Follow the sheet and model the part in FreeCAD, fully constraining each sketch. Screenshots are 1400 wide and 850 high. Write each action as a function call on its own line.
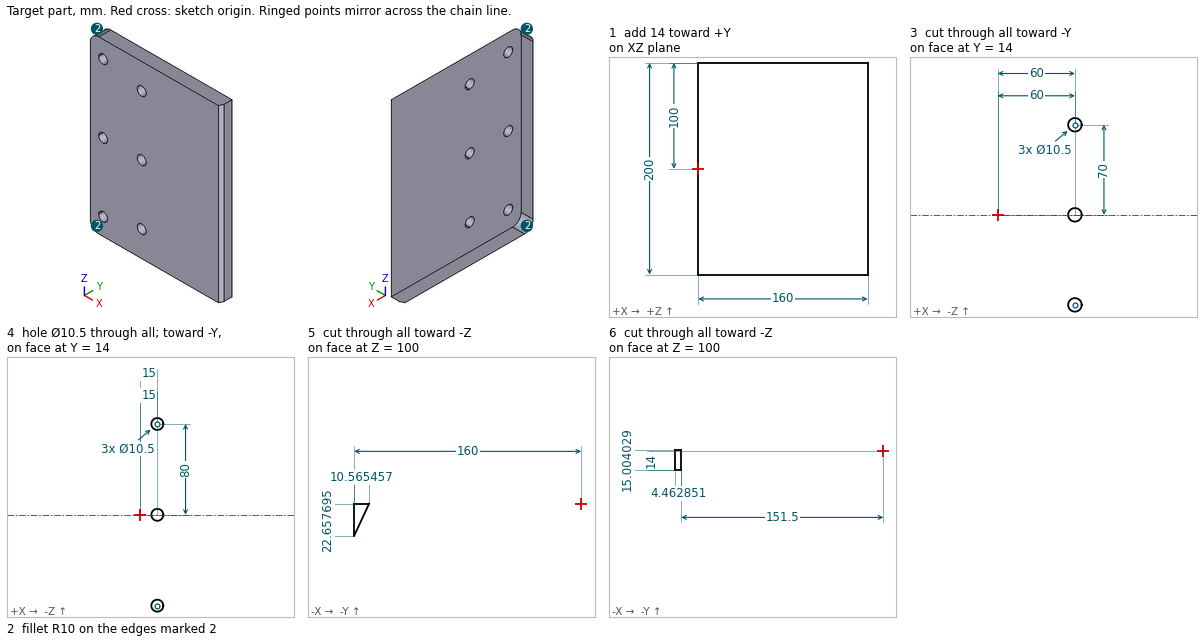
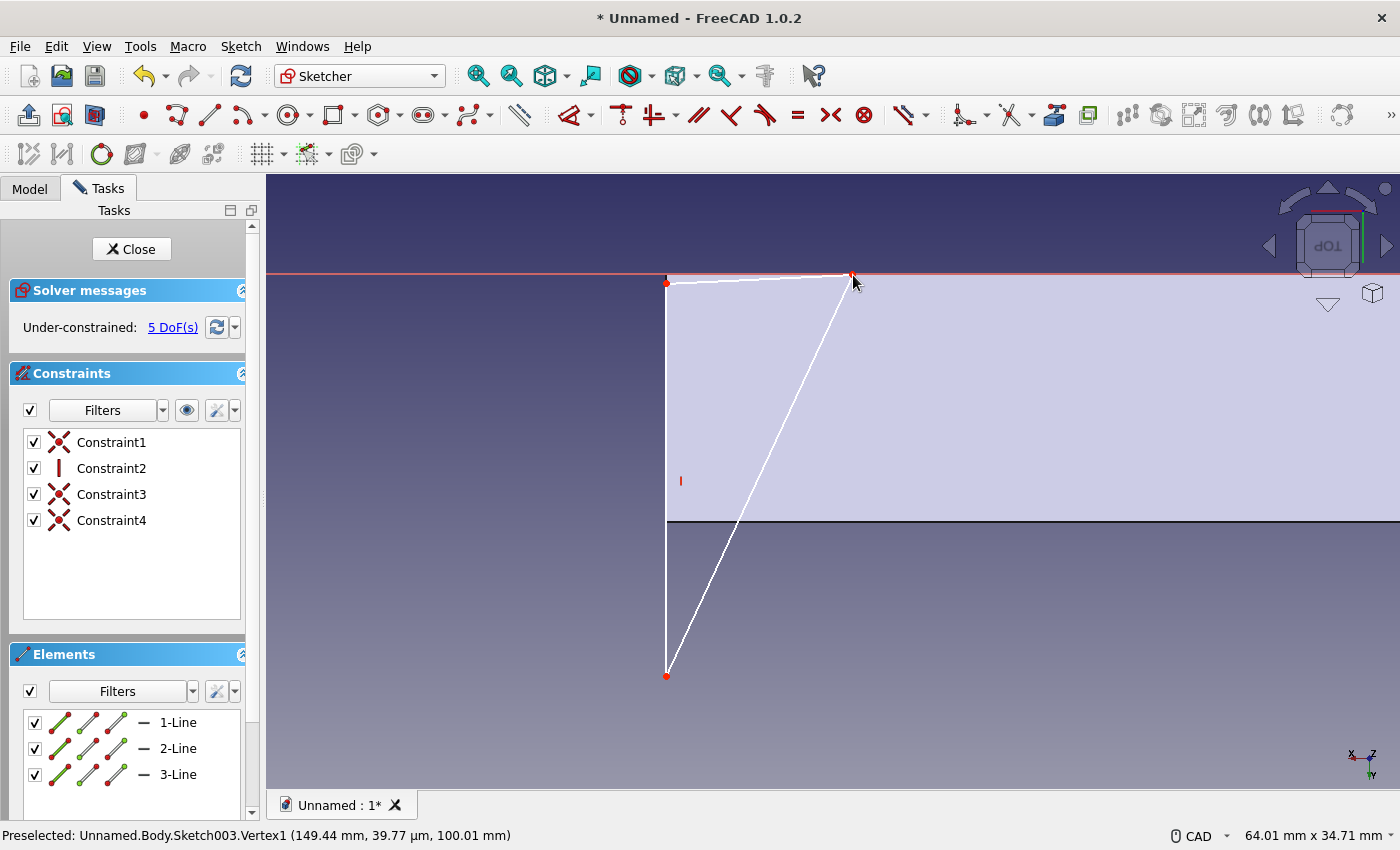
click(797, 278)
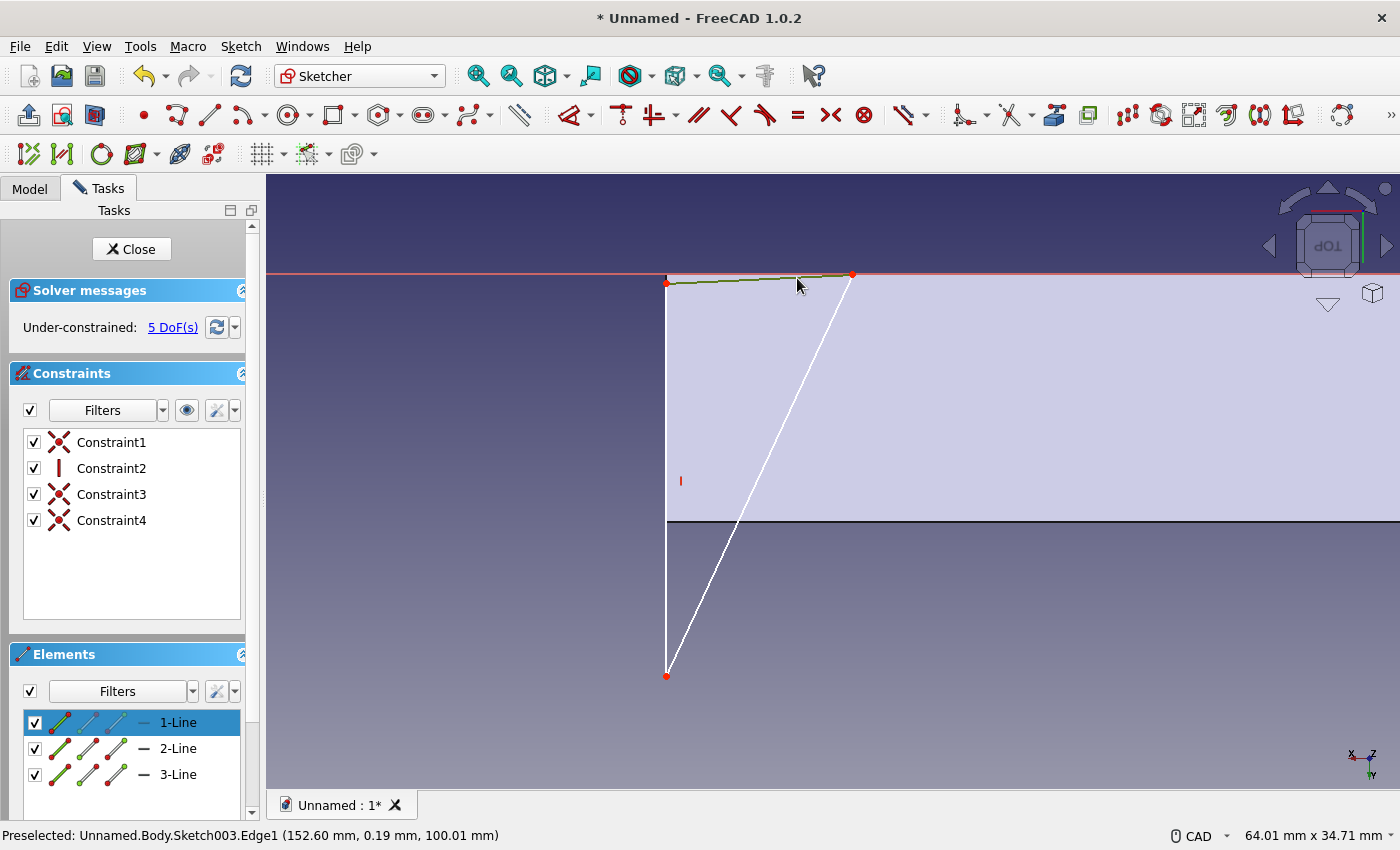
key(h)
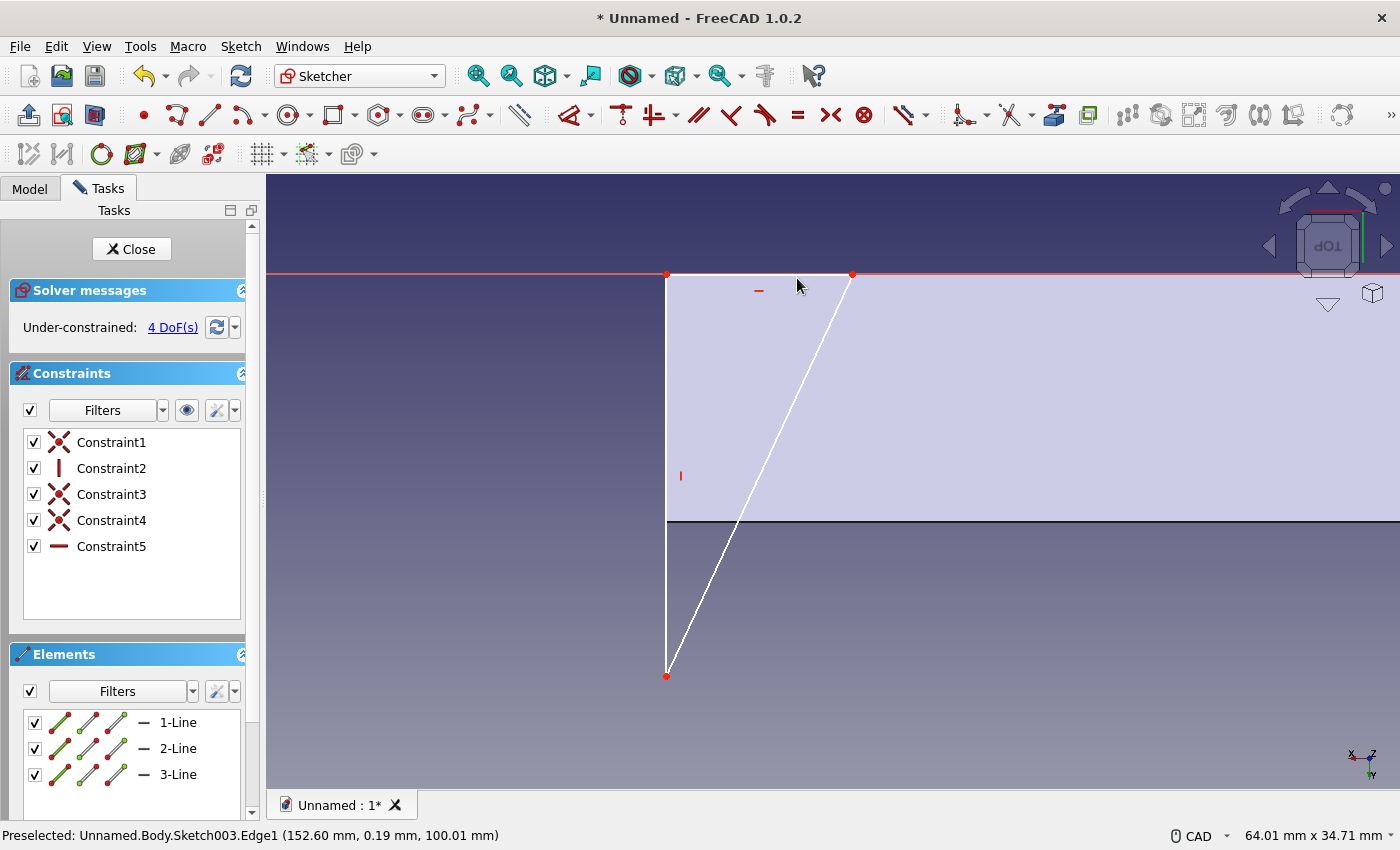
click(853, 275)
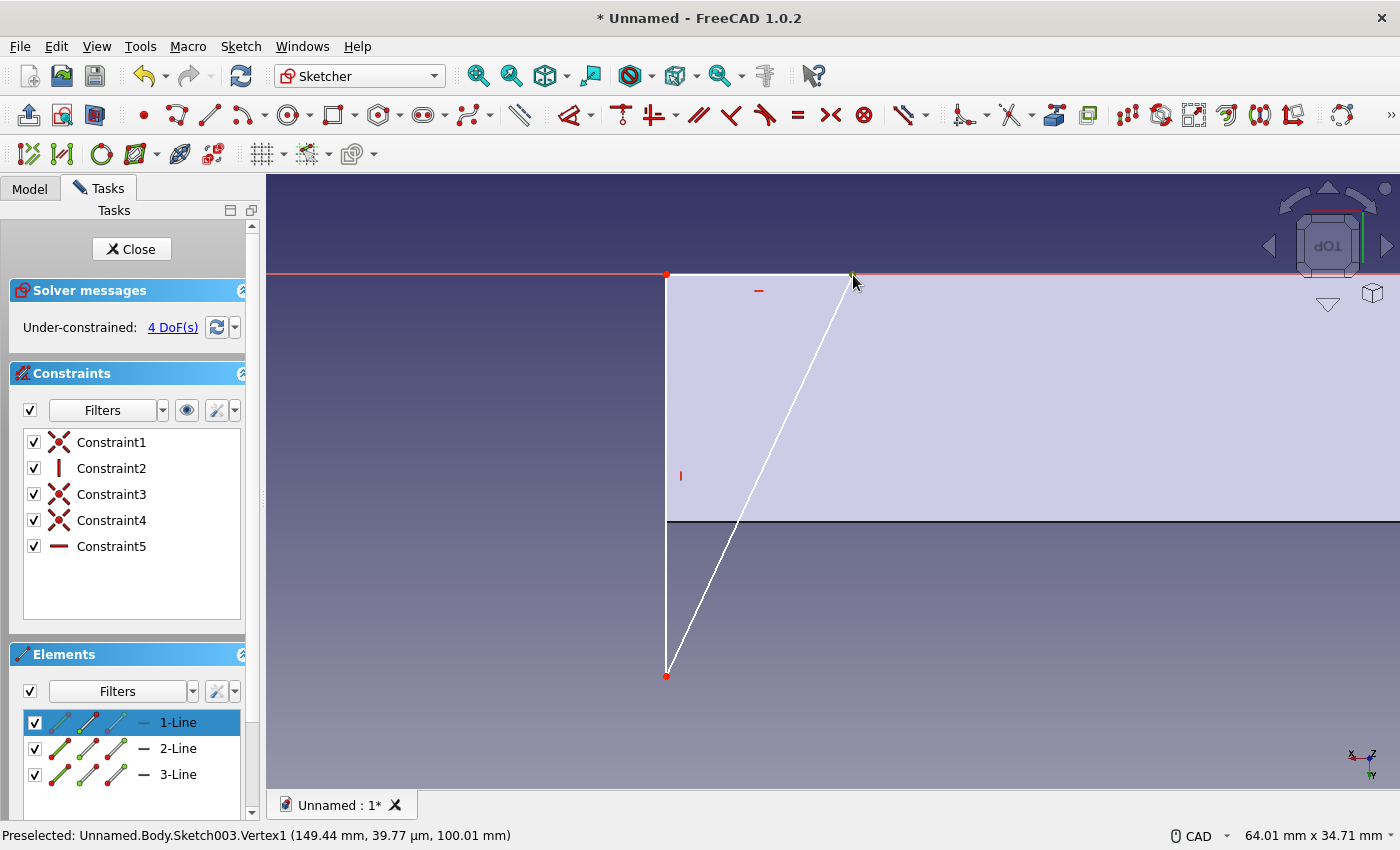
click(361, 274)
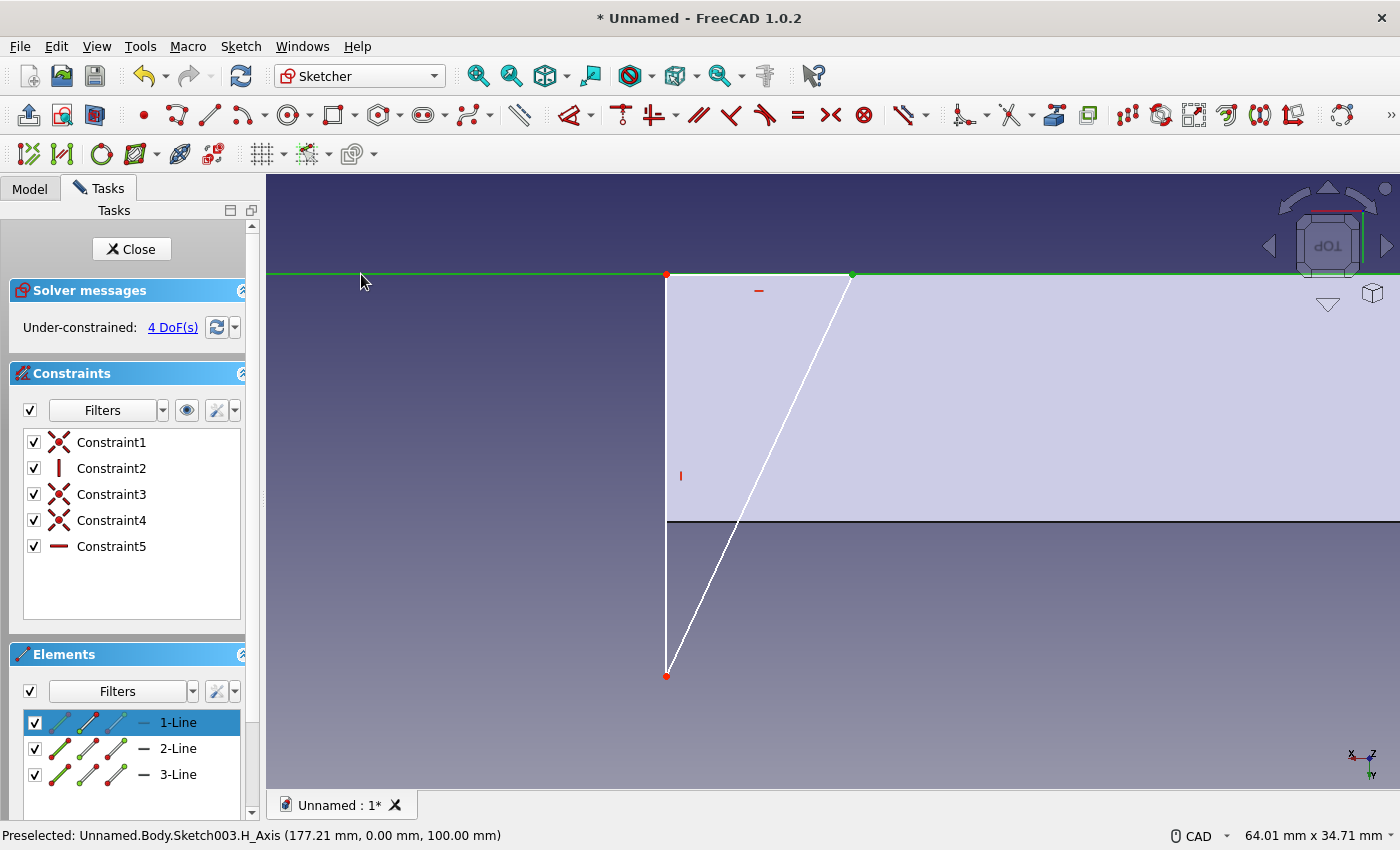
click(621, 116)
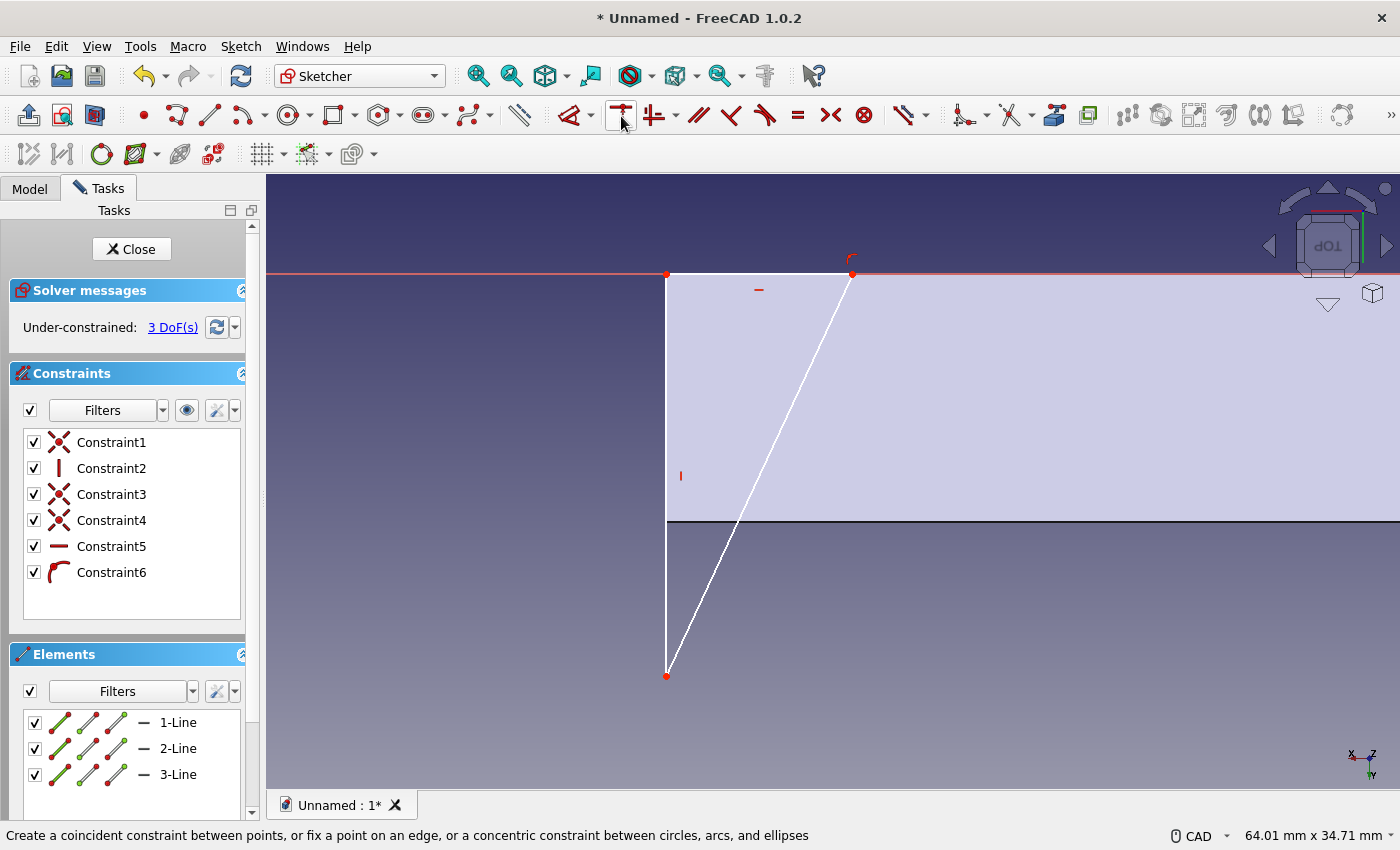
click(568, 116)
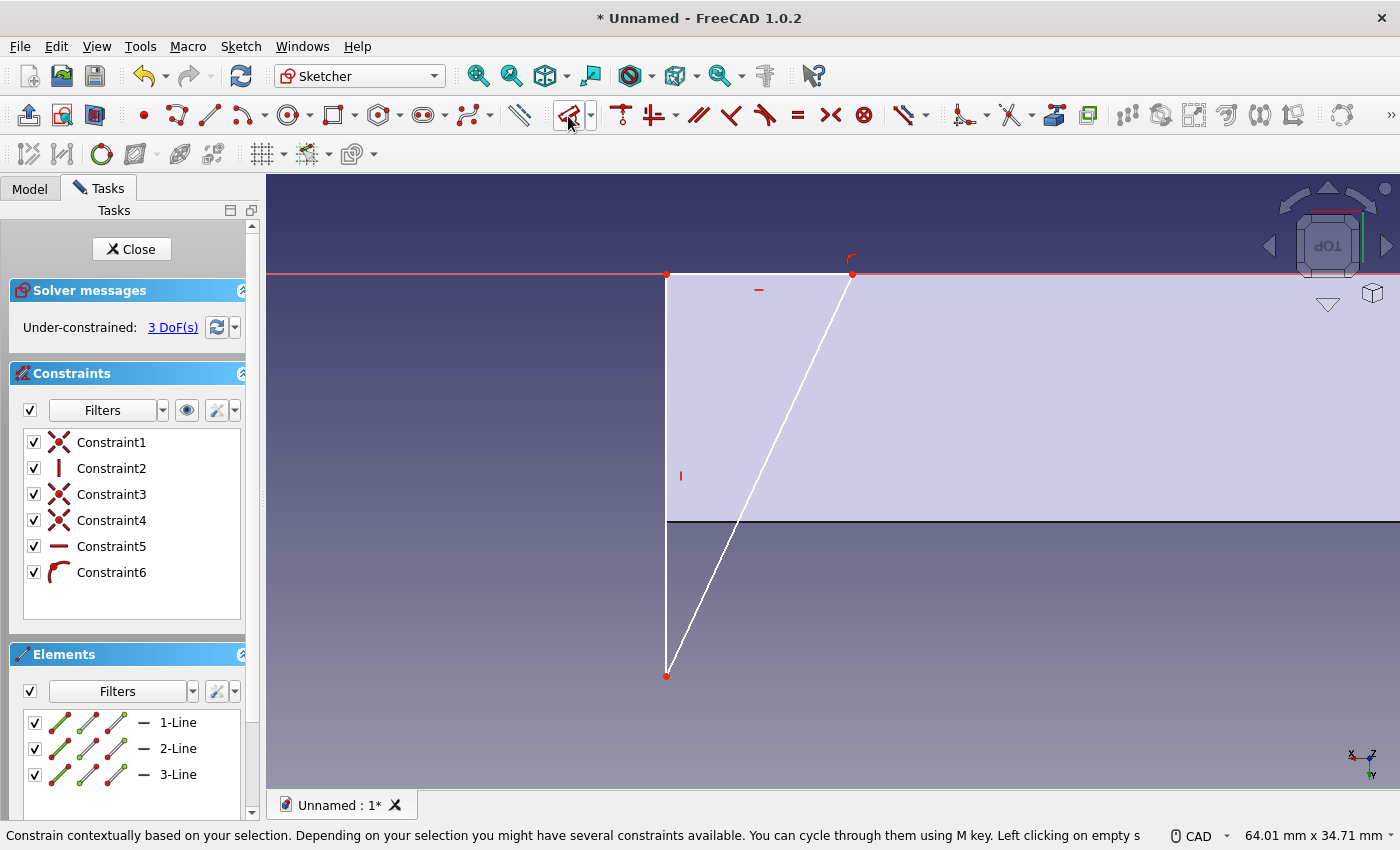
click(666, 274)
click(950, 240)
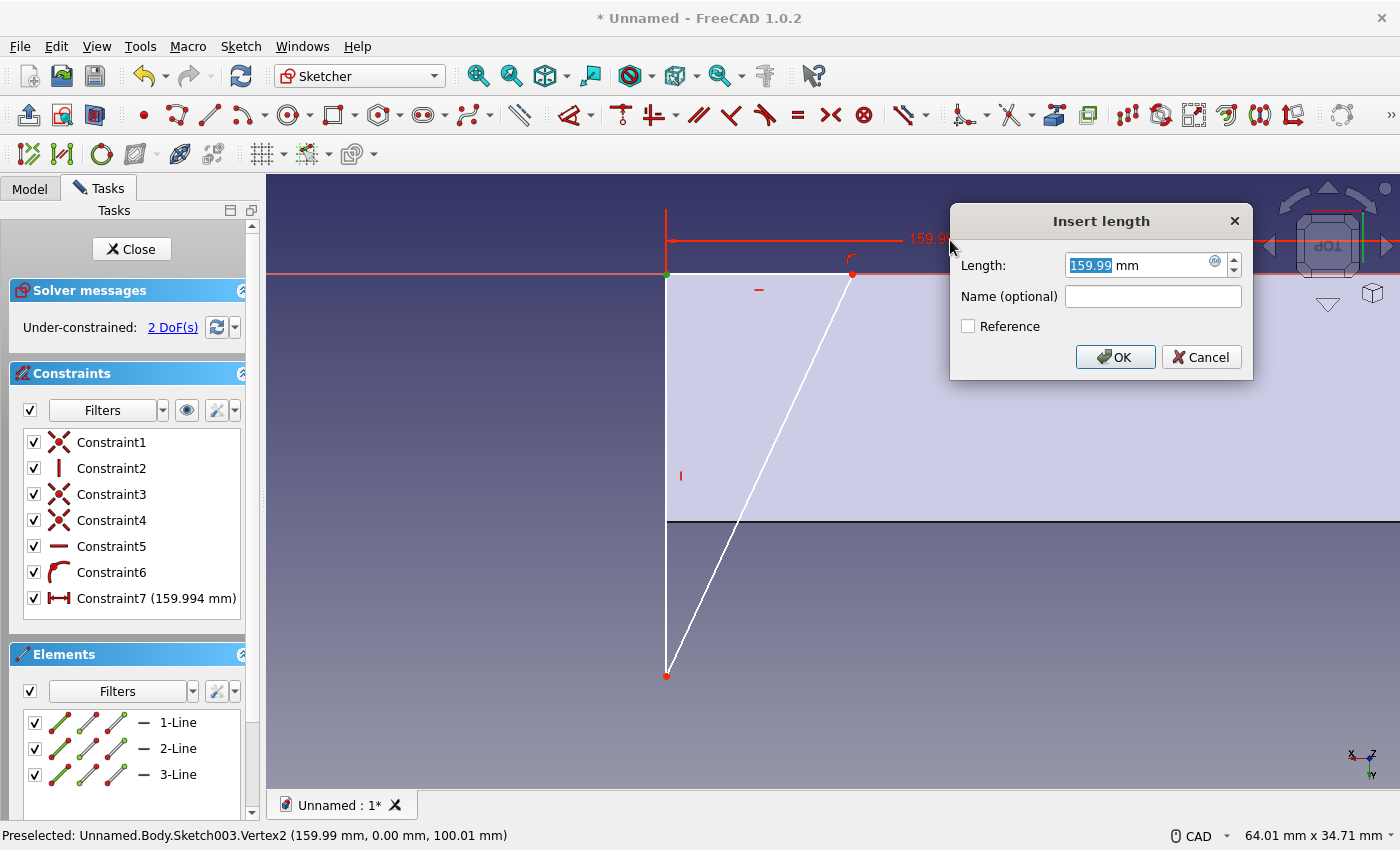
text(160)
key(Return)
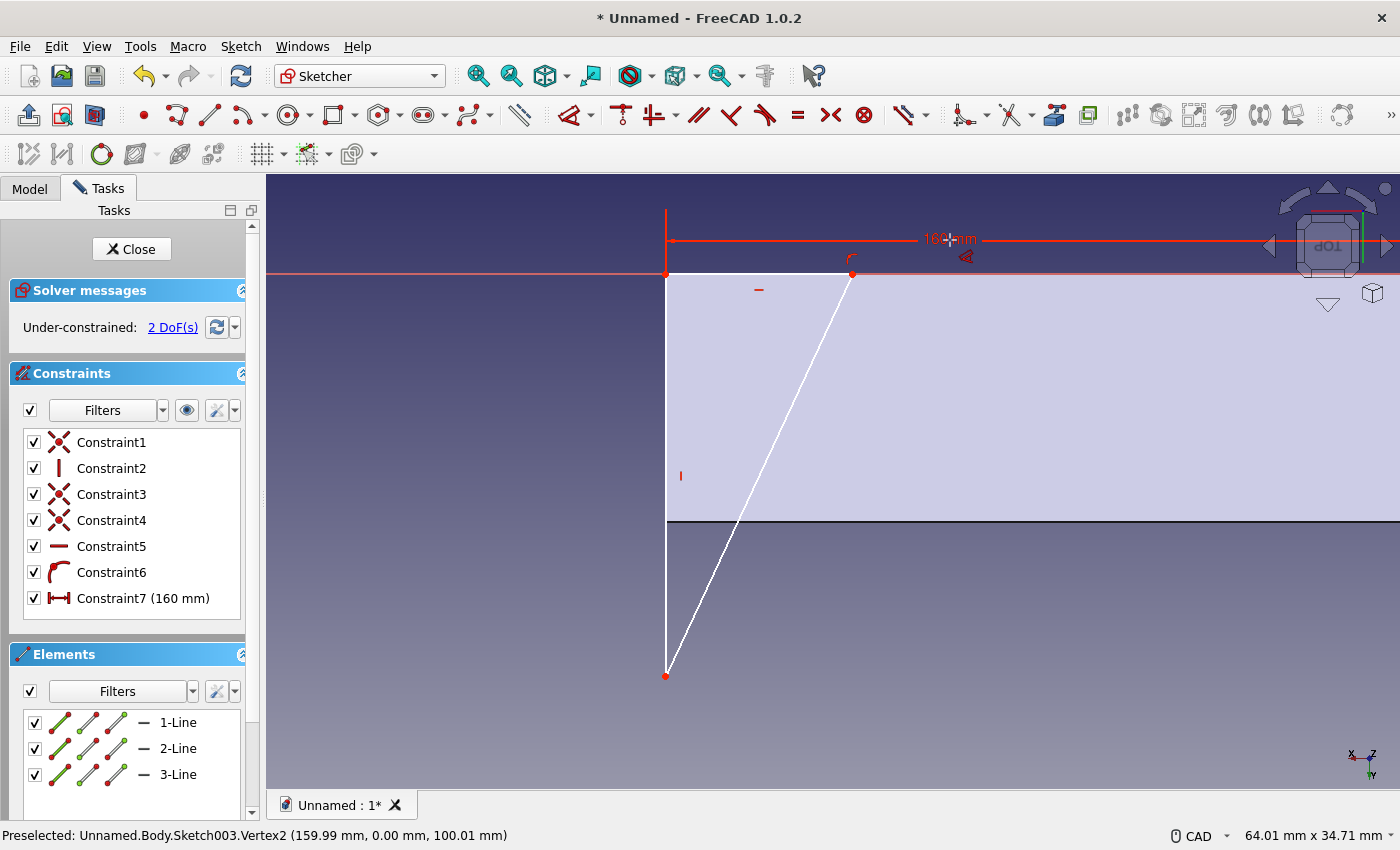
click(797, 274)
click(759, 240)